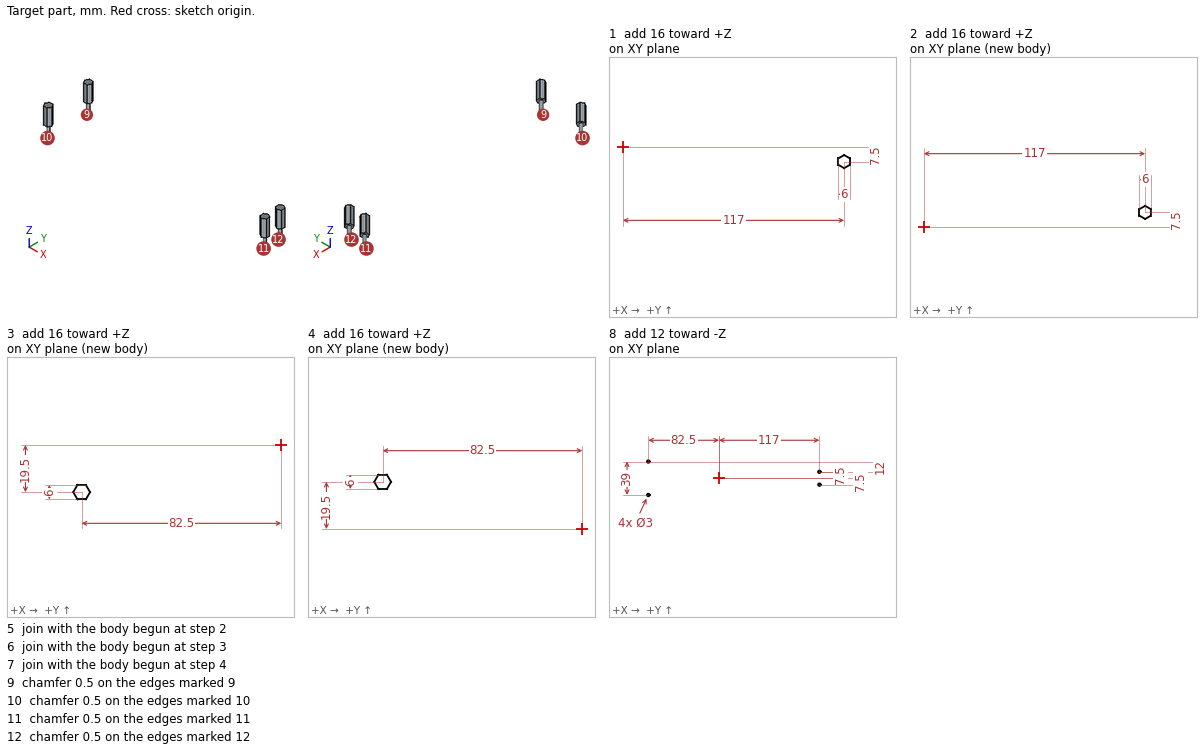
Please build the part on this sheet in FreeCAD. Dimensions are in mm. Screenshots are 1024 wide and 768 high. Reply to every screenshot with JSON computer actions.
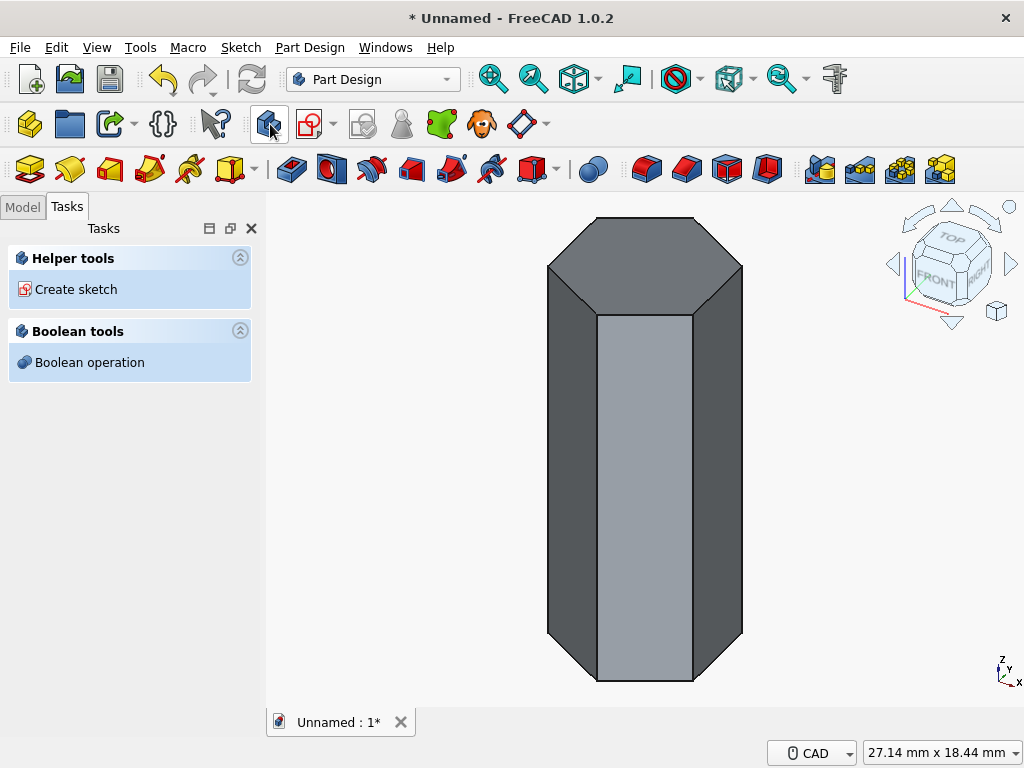
{"action": "left_click", "coordinate": [306, 667]}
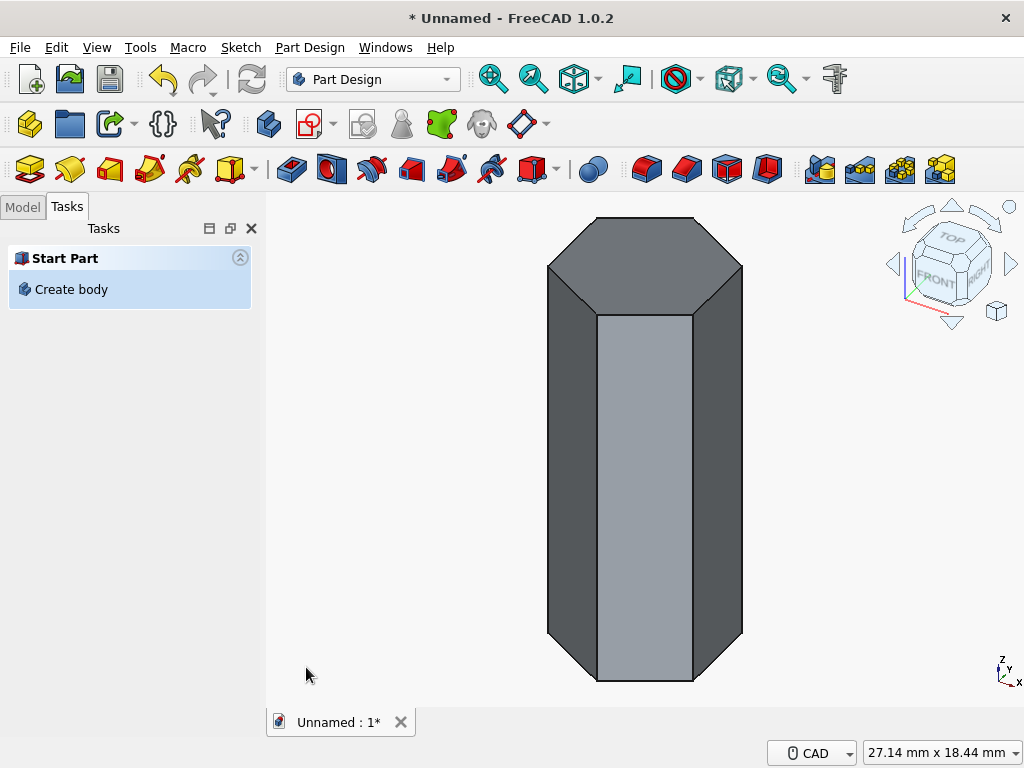
{"action": "left_click", "coordinate": [310, 124]}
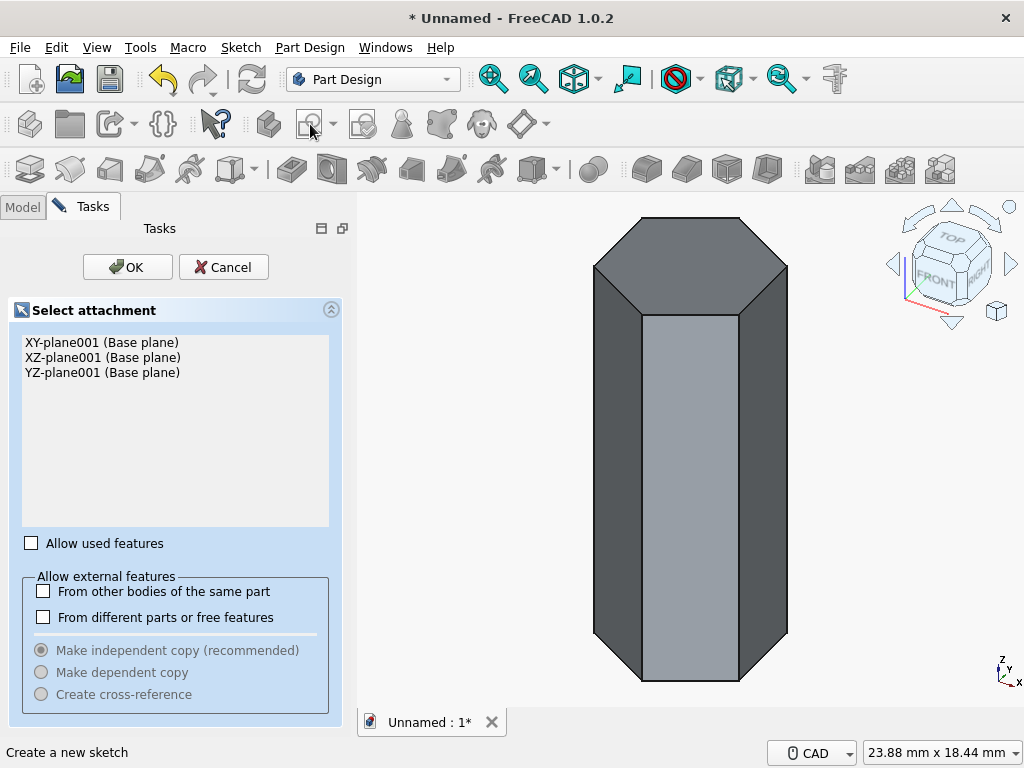
{"action": "left_click", "coordinate": [82, 342]}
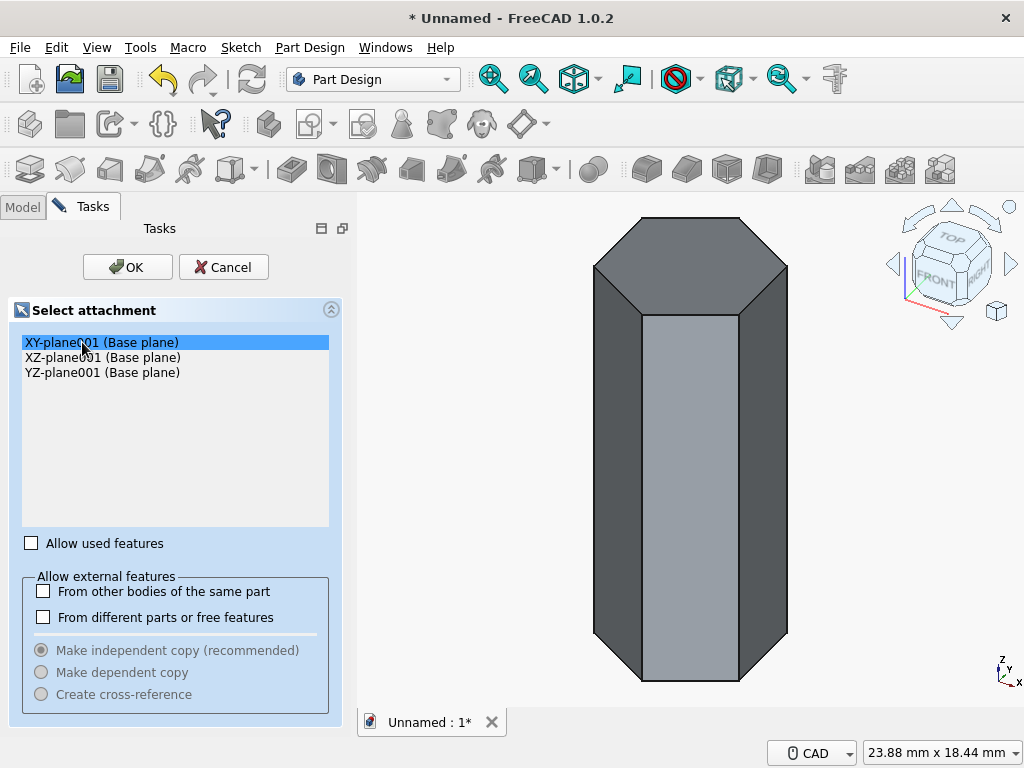
{"action": "left_click", "coordinate": [128, 267]}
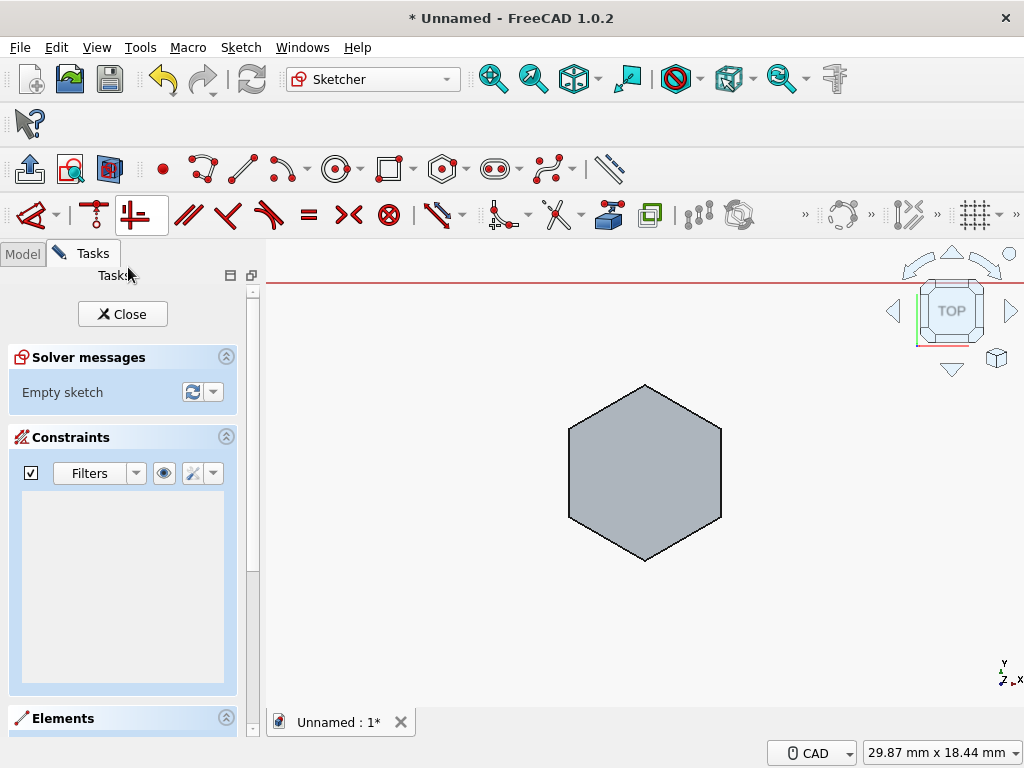
{"action": "scroll", "coordinate": [576, 473], "scroll_direction": "down", "scroll_amount": 5}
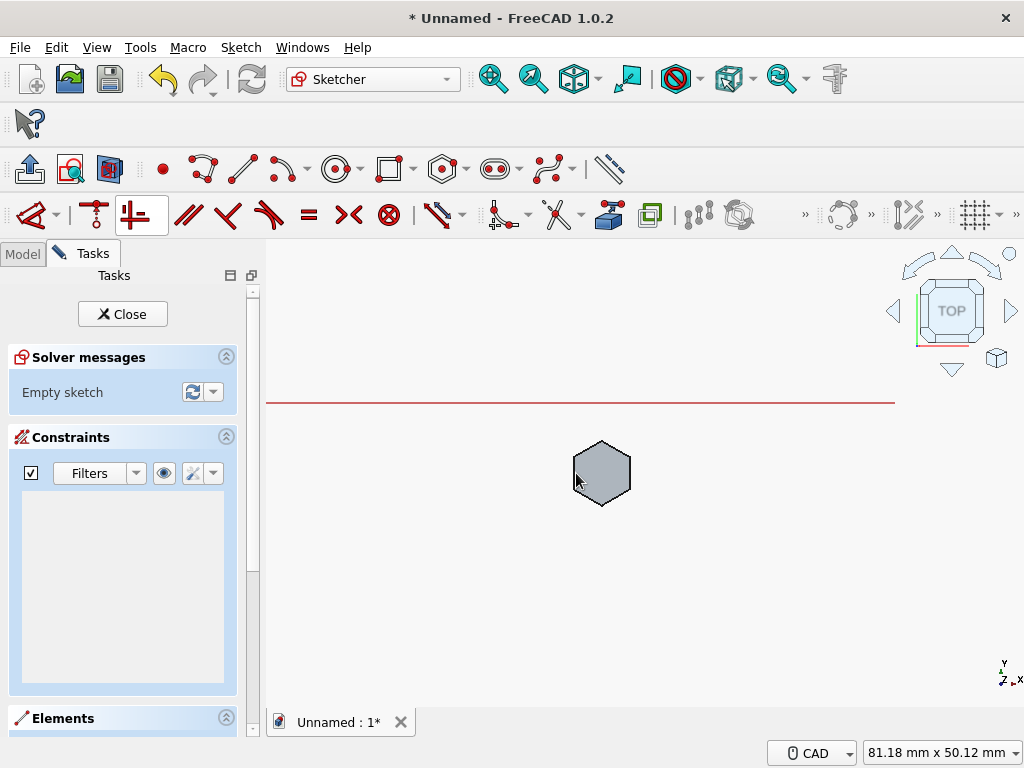
{"action": "scroll", "coordinate": [608, 298], "scroll_direction": "up", "scroll_amount": 8}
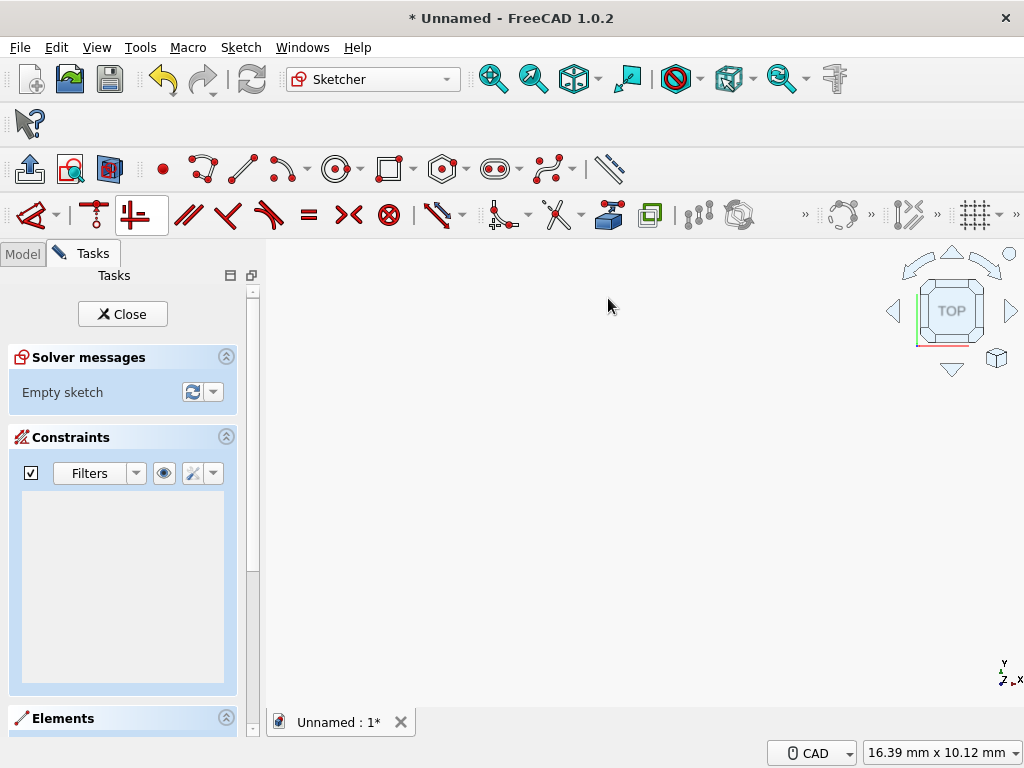
{"action": "left_click", "coordinate": [442, 170]}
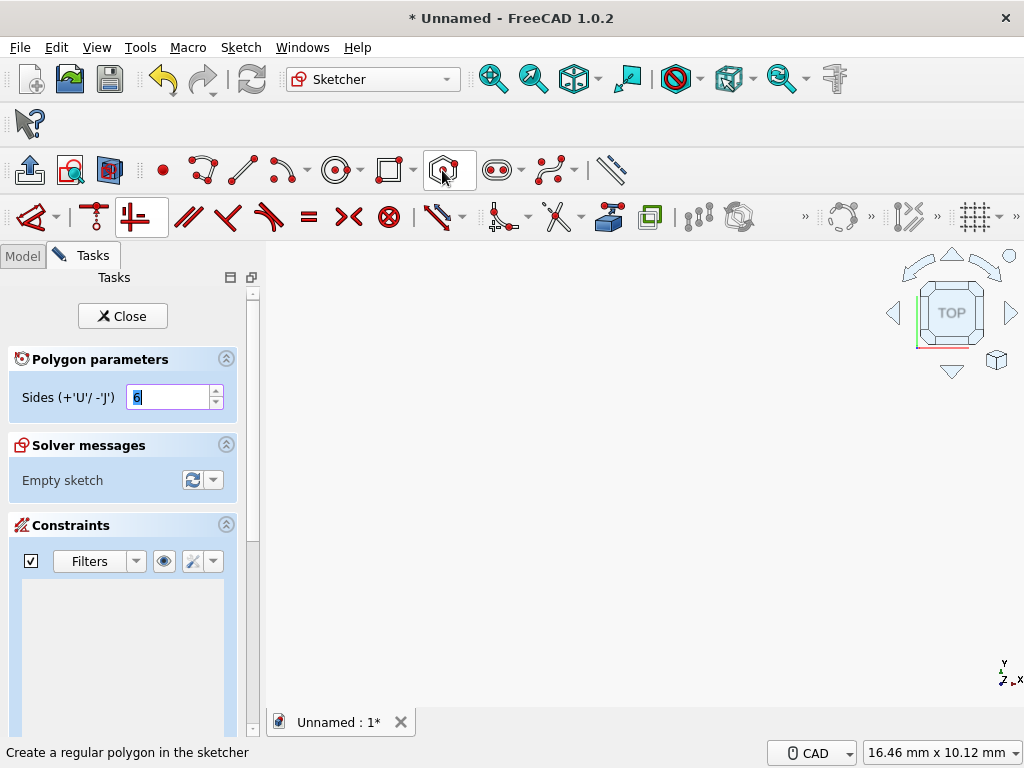
{"action": "left_click", "coordinate": [575, 473]}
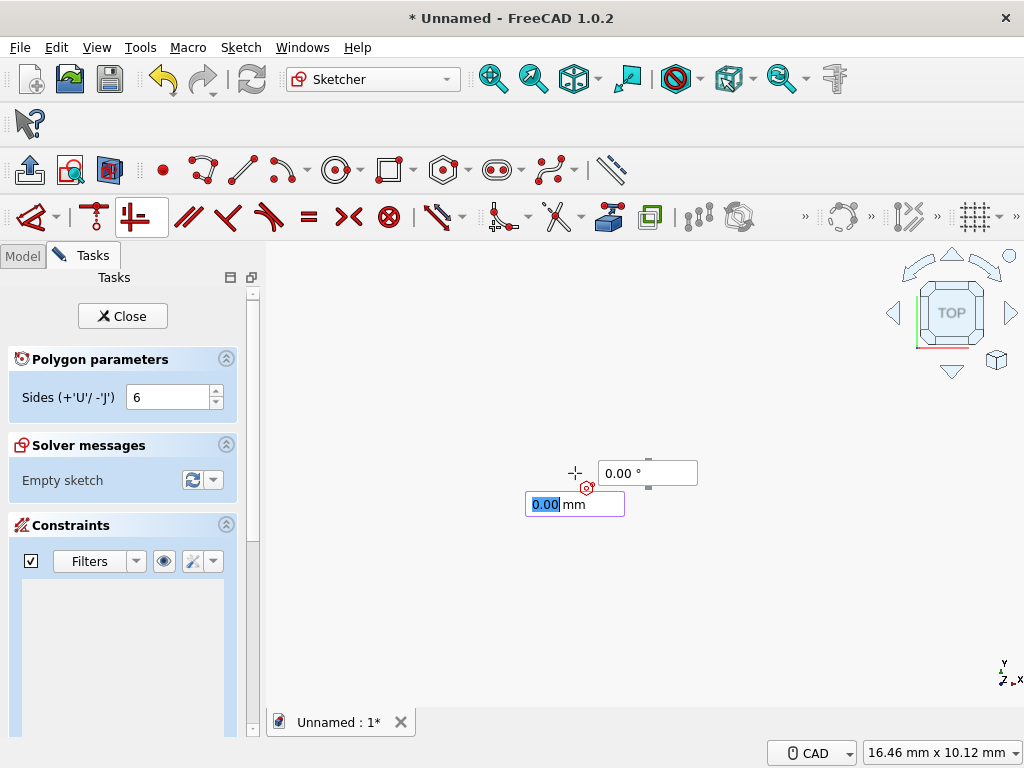
{"action": "left_click", "coordinate": [575, 314]}
{"action": "right_click", "coordinate": [575, 314]}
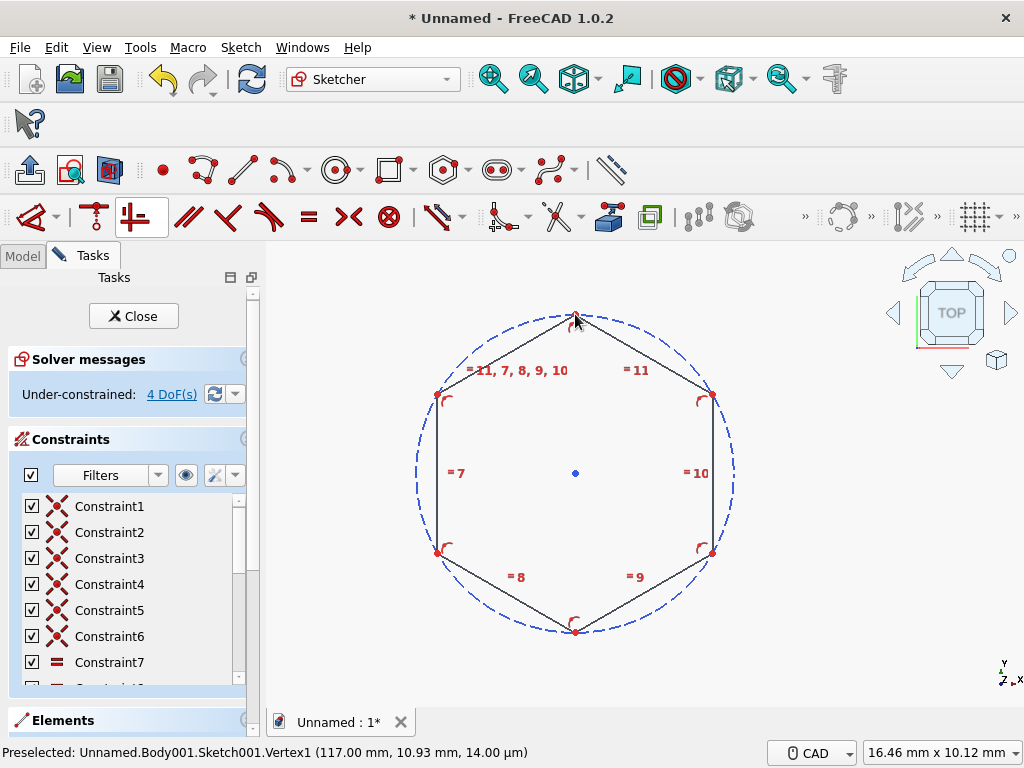
{"action": "left_click", "coordinate": [437, 442]}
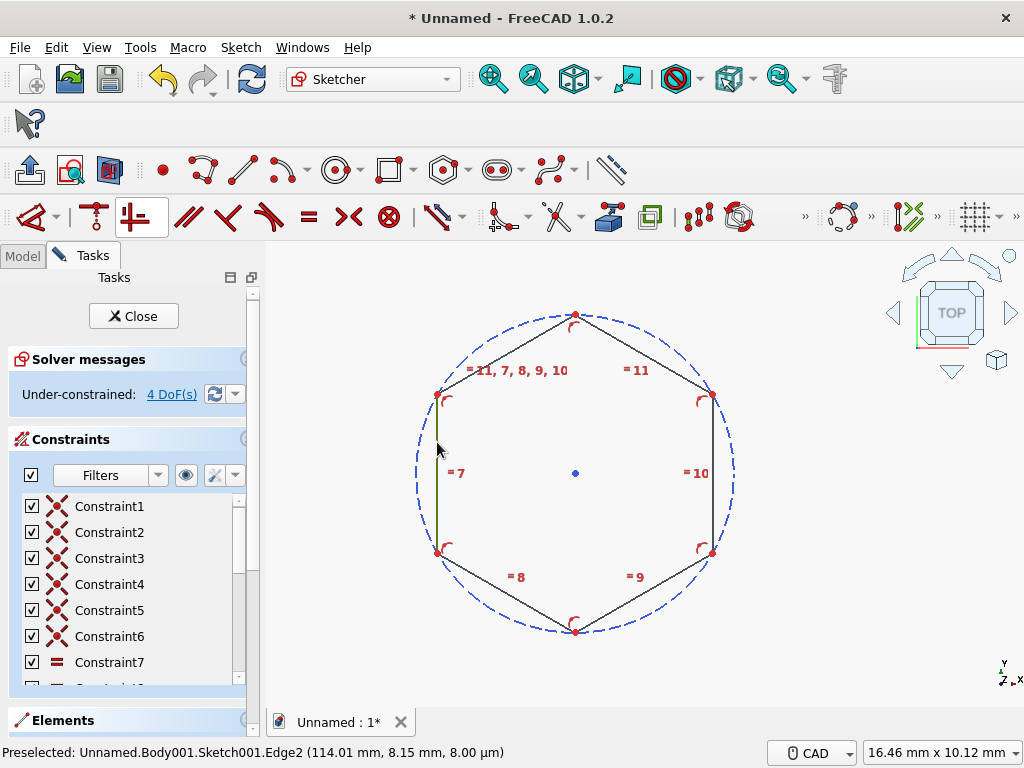
{"action": "left_click", "coordinate": [162, 218]}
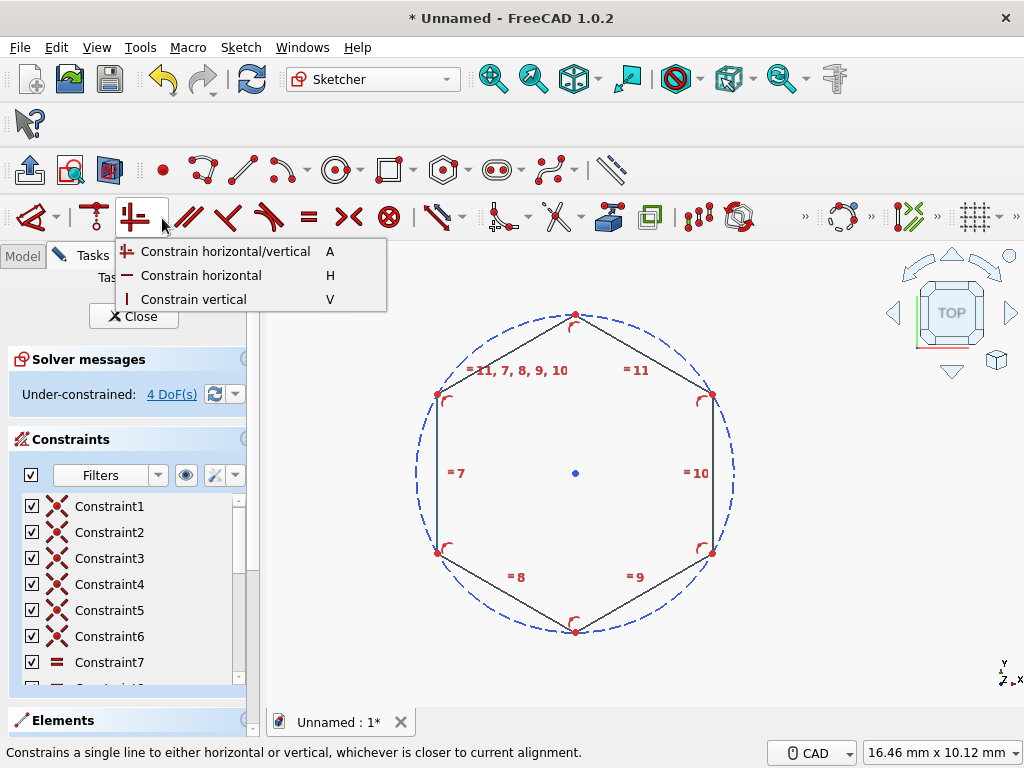
{"action": "left_click", "coordinate": [251, 299]}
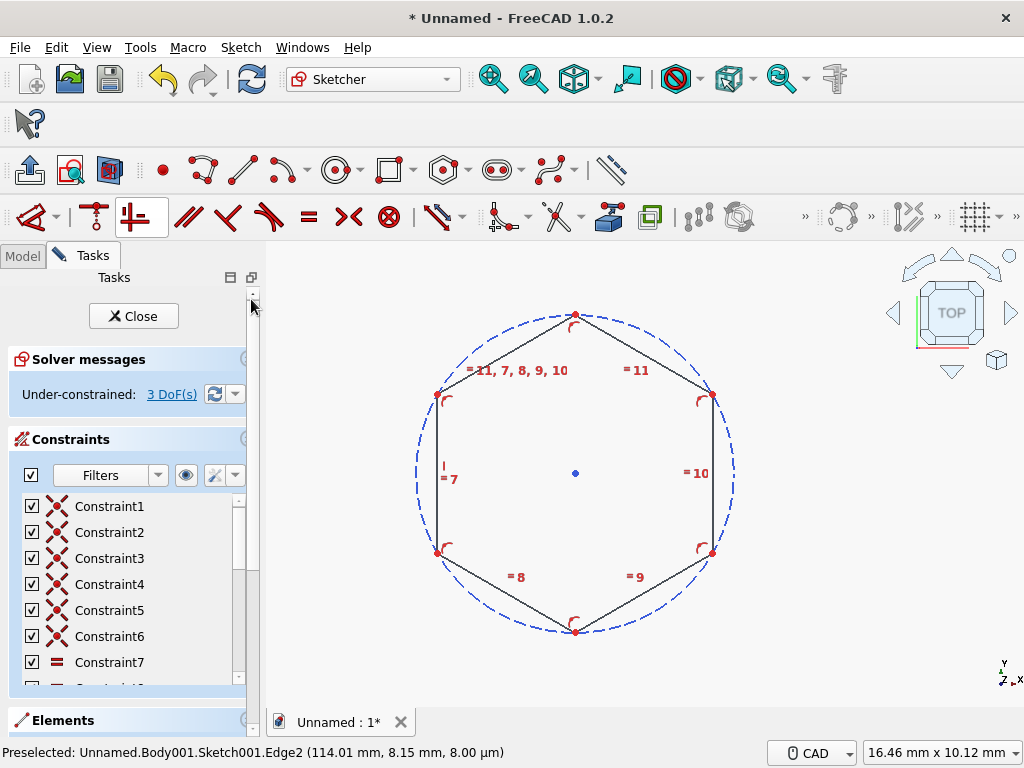
{"action": "left_click", "coordinate": [32, 218]}